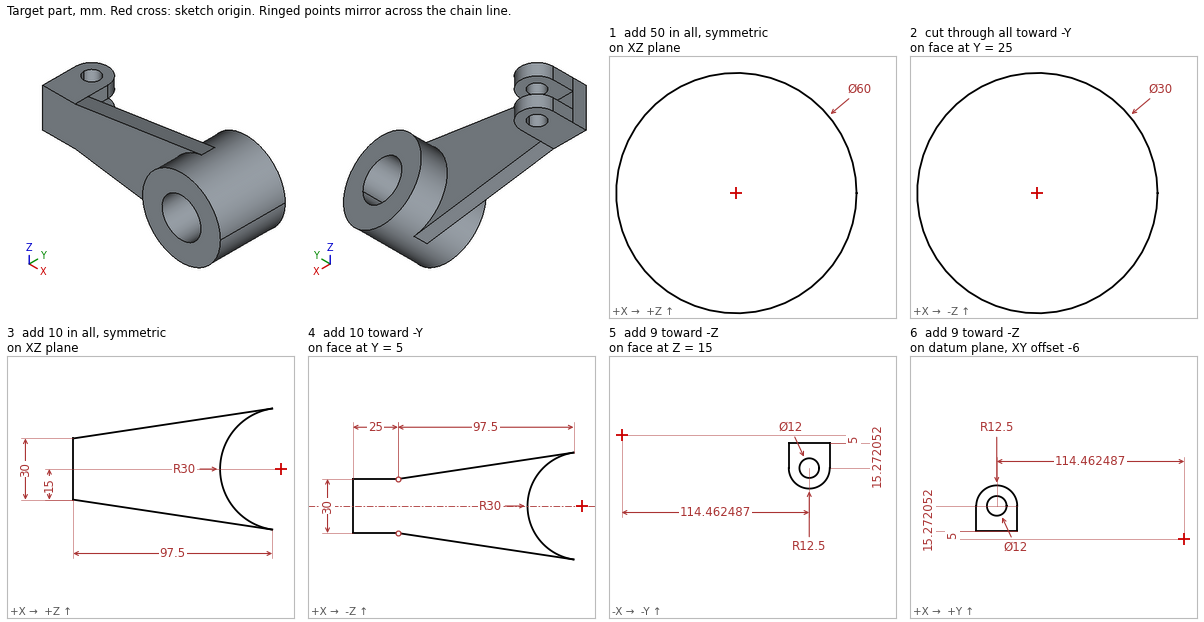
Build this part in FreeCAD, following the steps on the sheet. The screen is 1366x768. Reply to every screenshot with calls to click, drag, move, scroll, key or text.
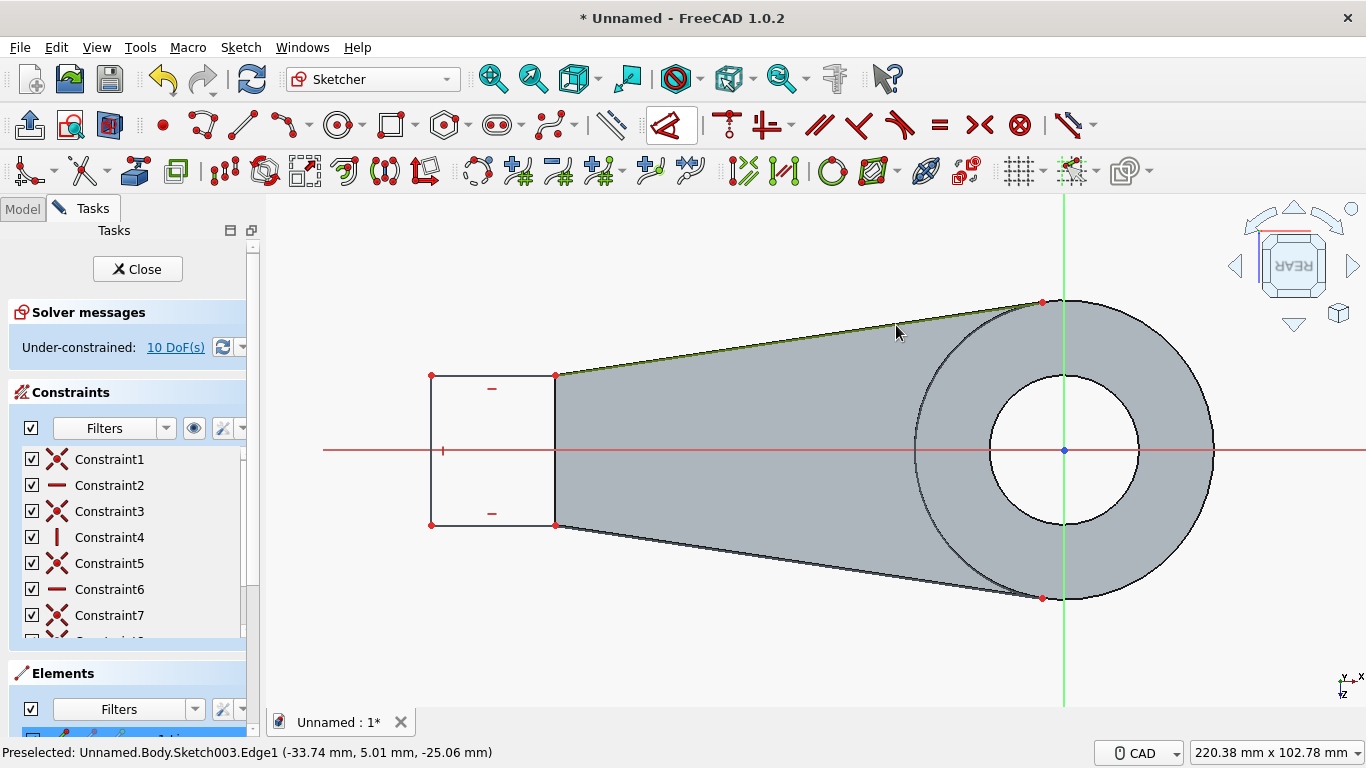
click(938, 371)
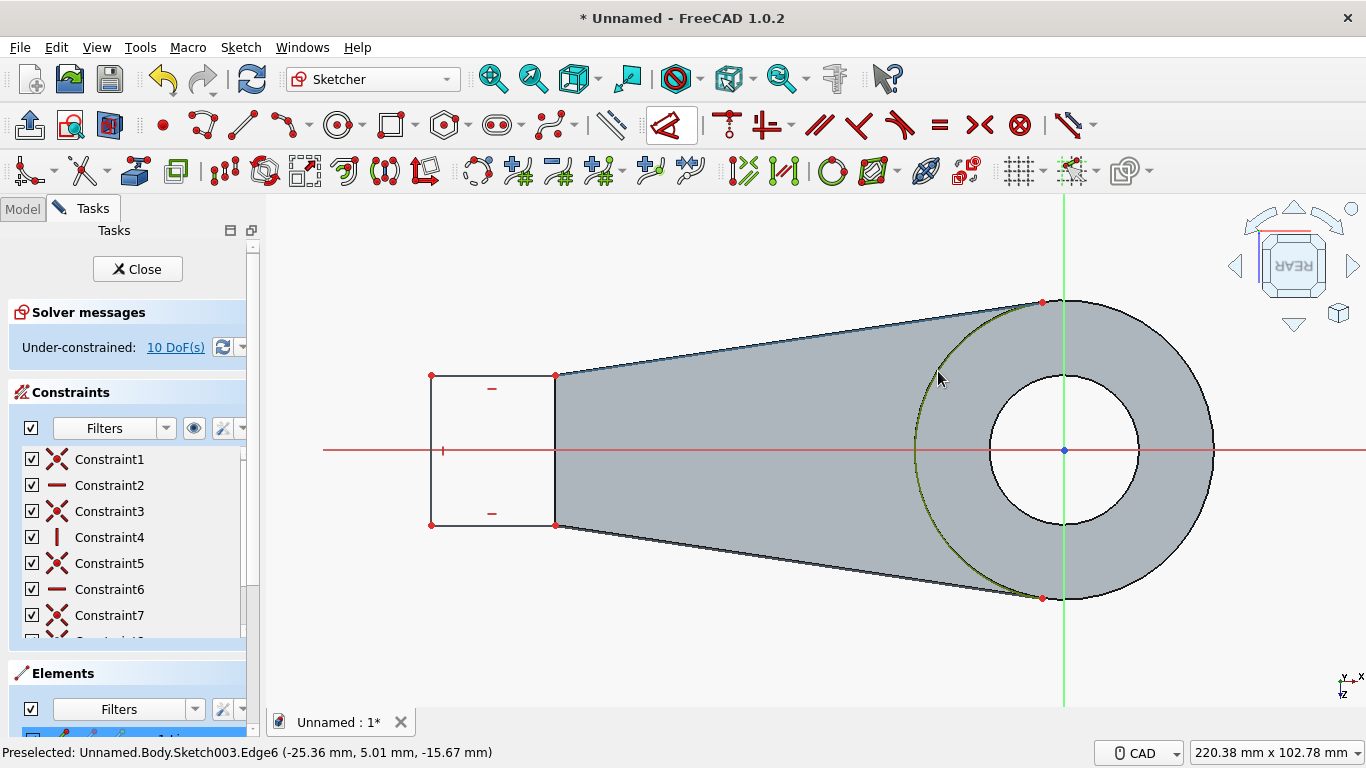
click(900, 126)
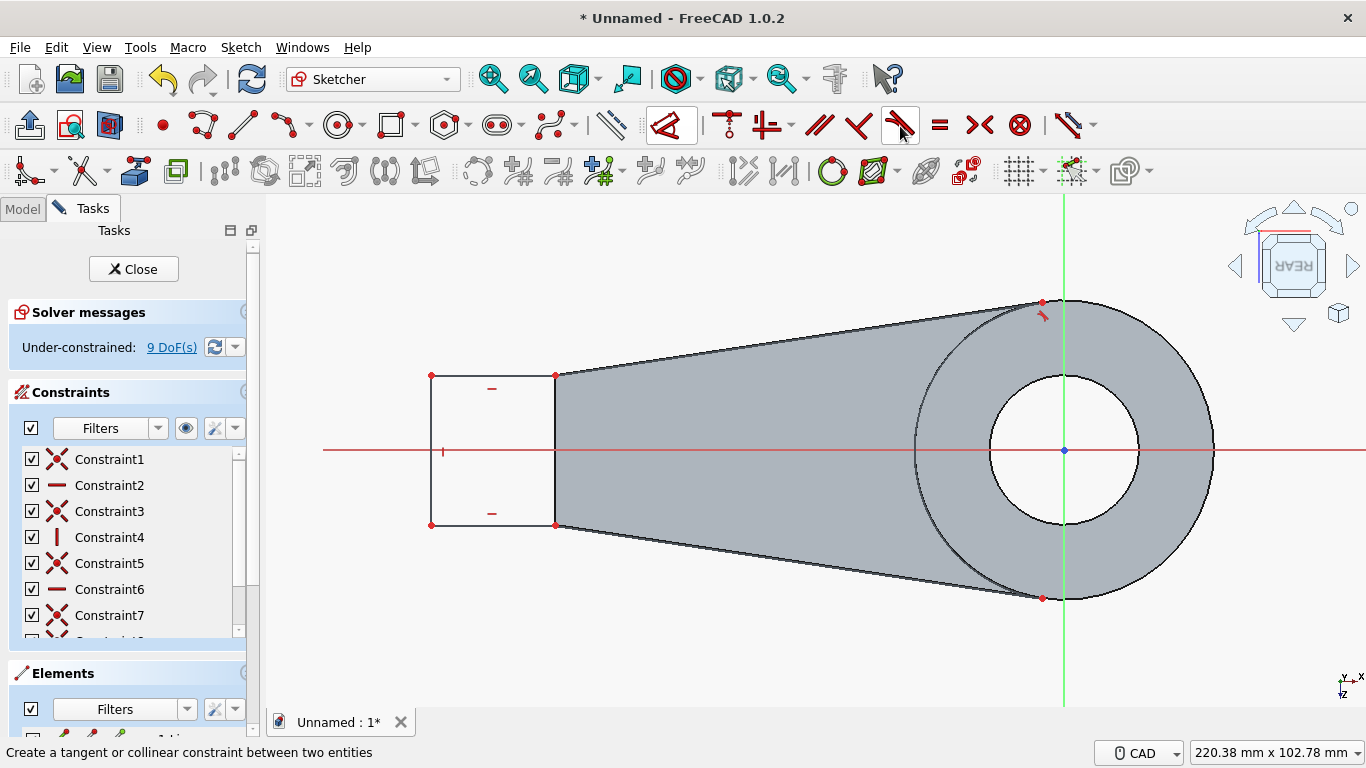
click(701, 548)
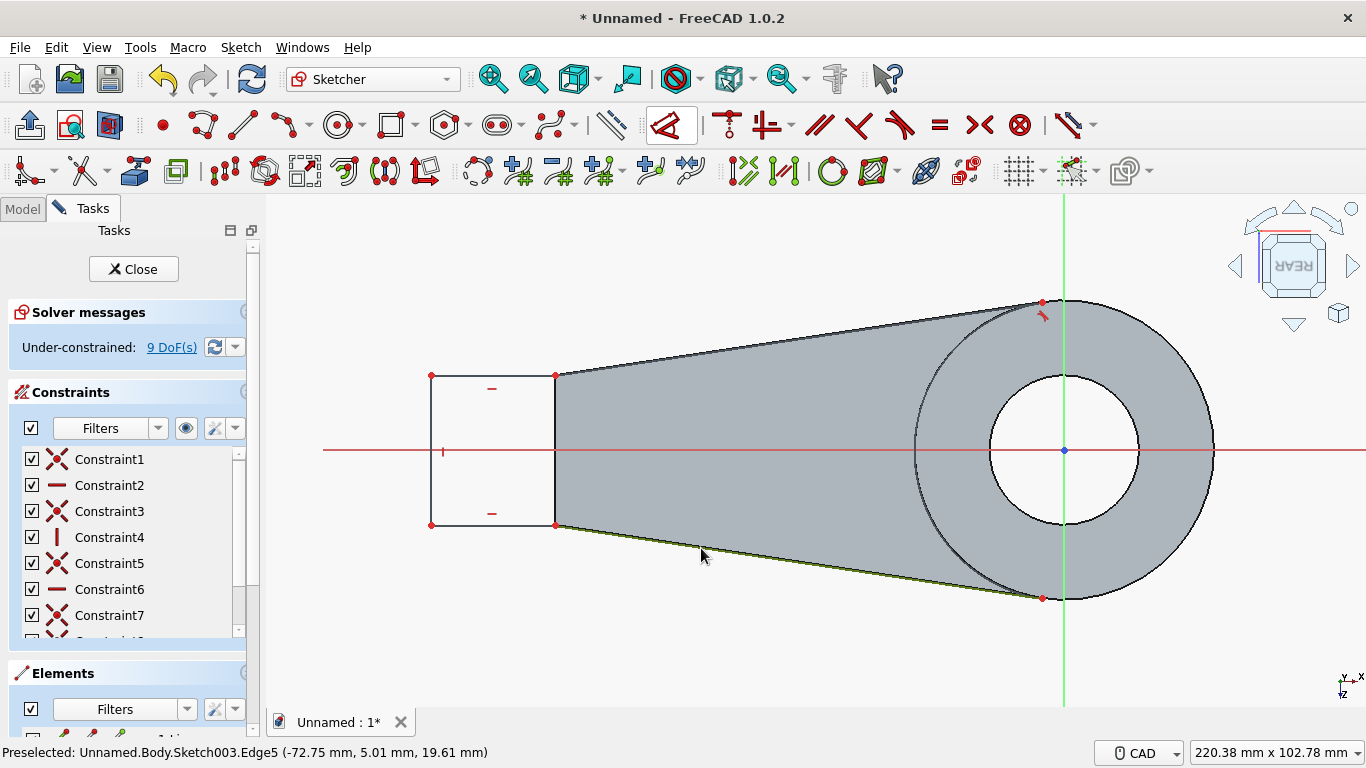
click(938, 370)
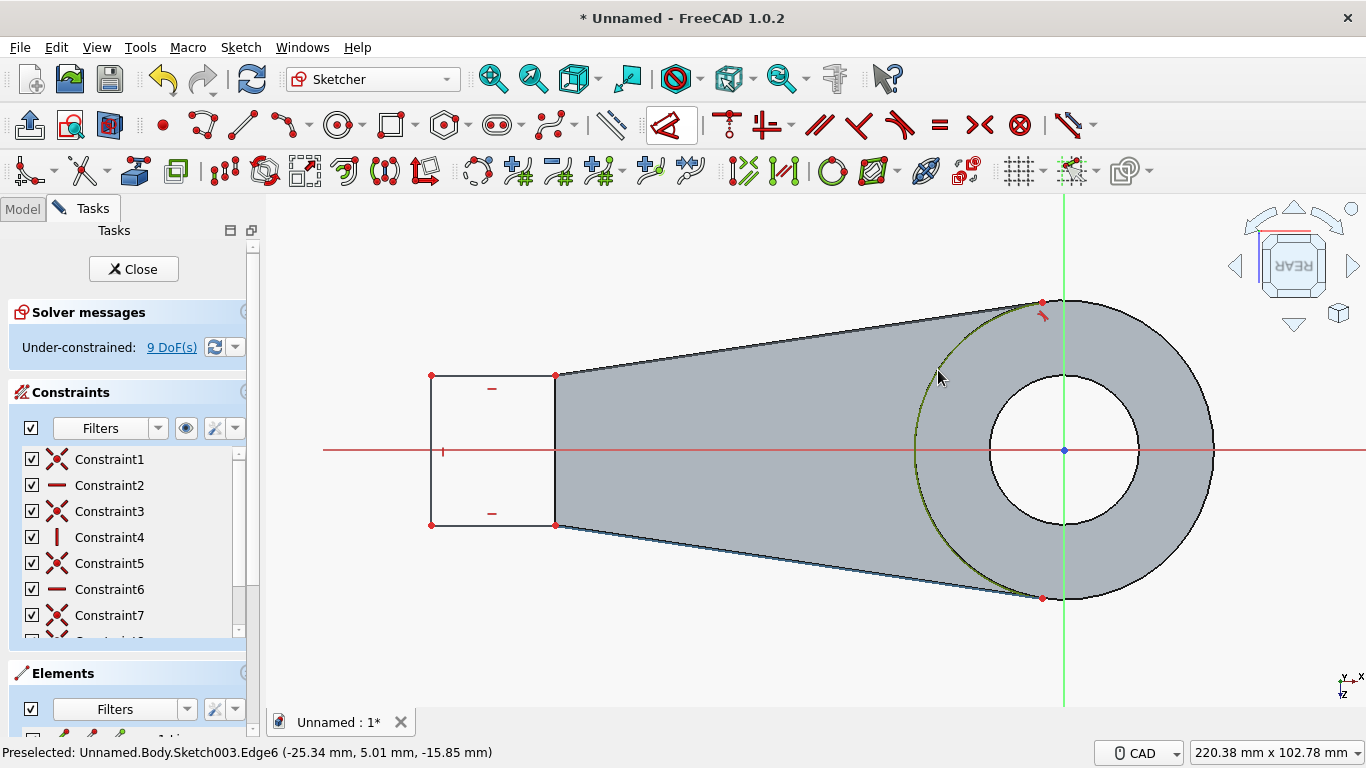
click(900, 126)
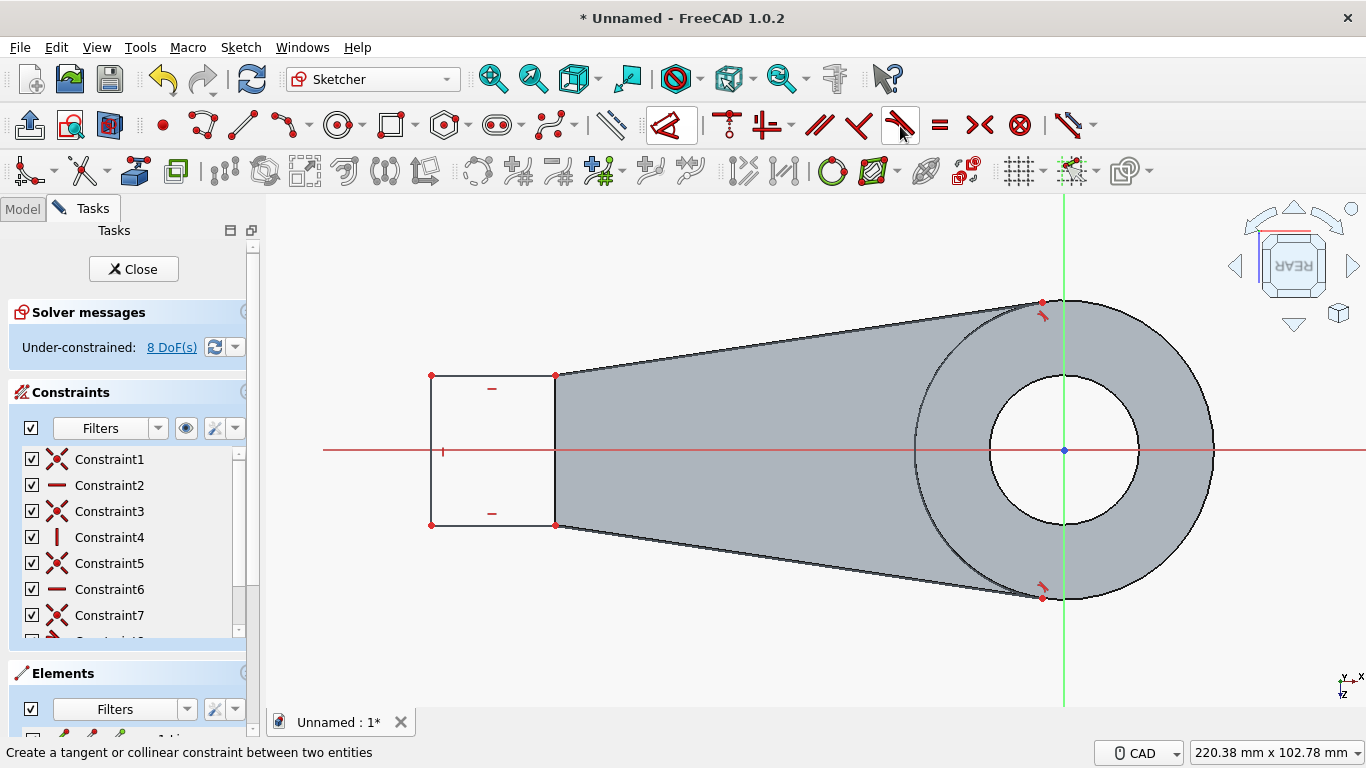
drag(1054, 440, 1074, 461)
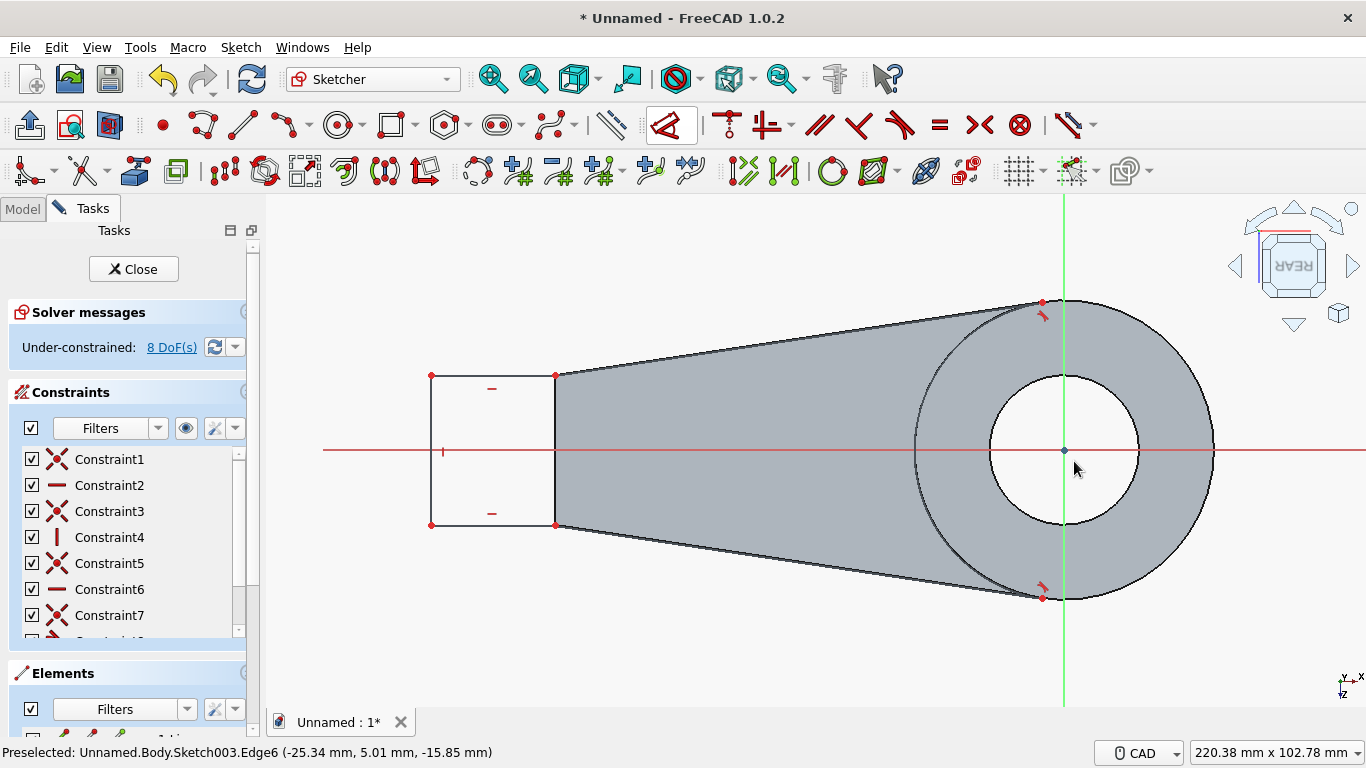
click(728, 126)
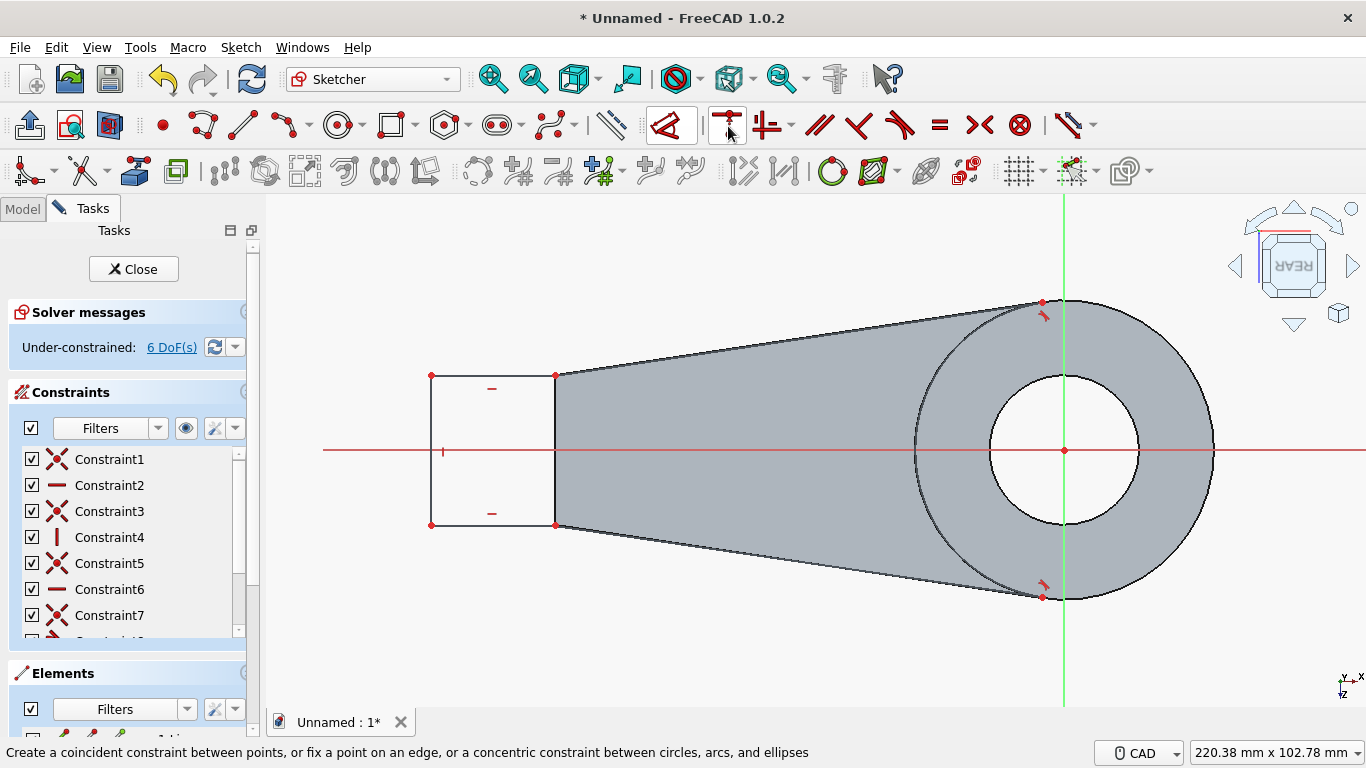
click(555, 376)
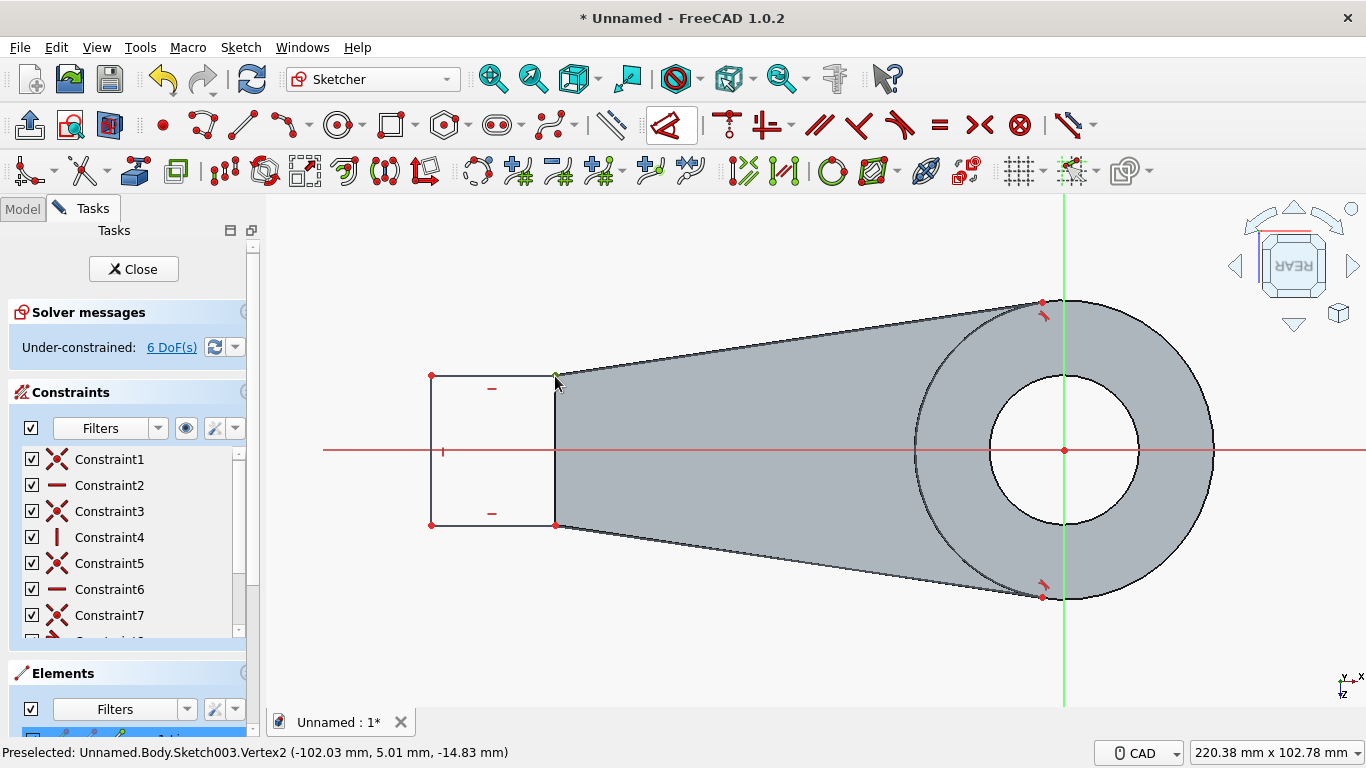
click(555, 526)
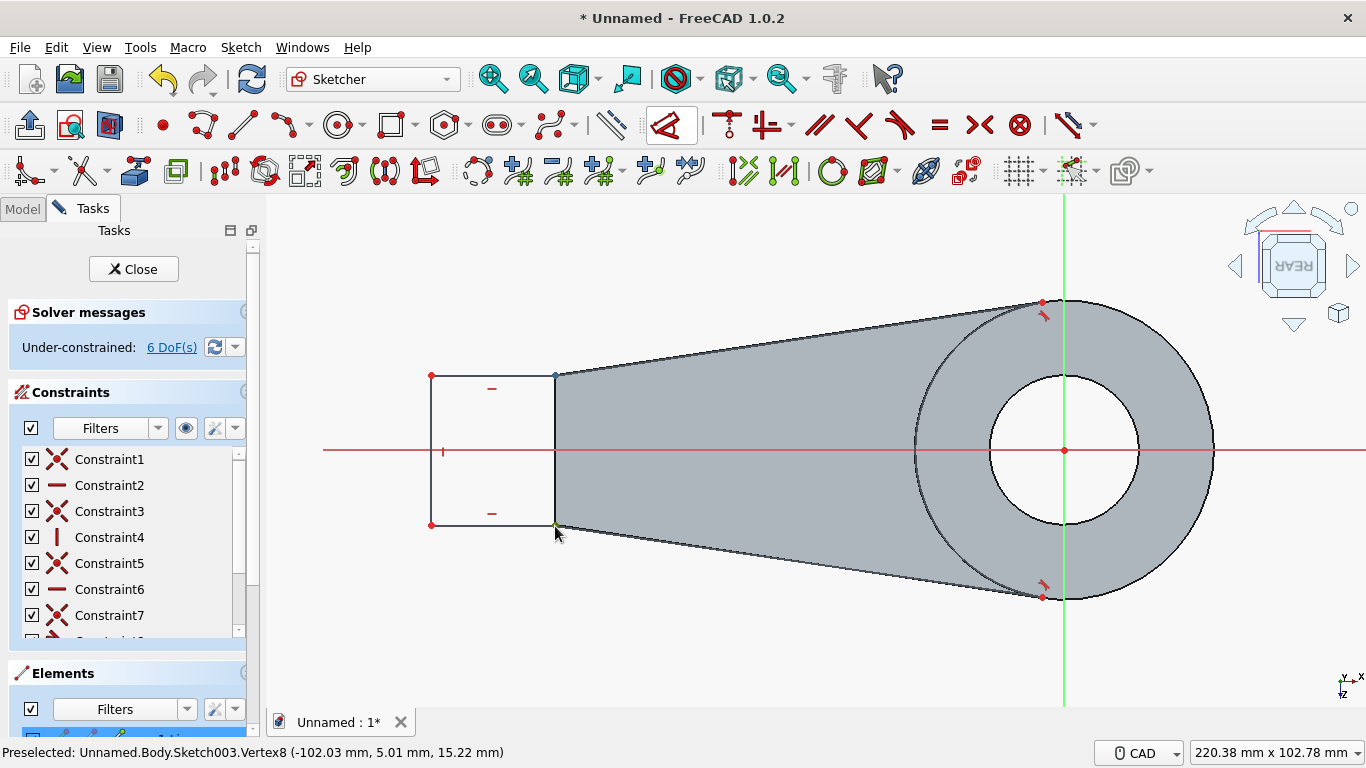
click(359, 450)